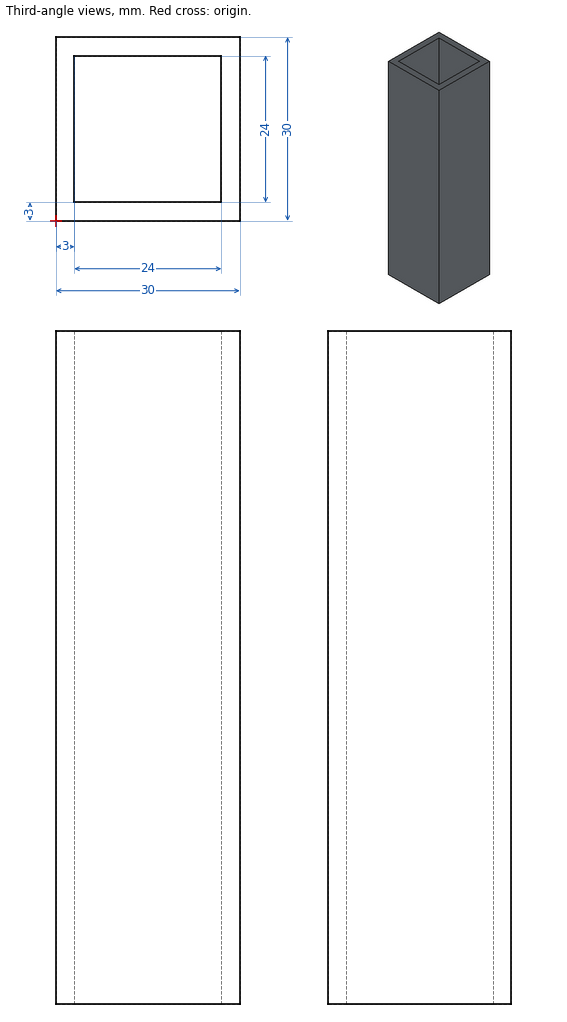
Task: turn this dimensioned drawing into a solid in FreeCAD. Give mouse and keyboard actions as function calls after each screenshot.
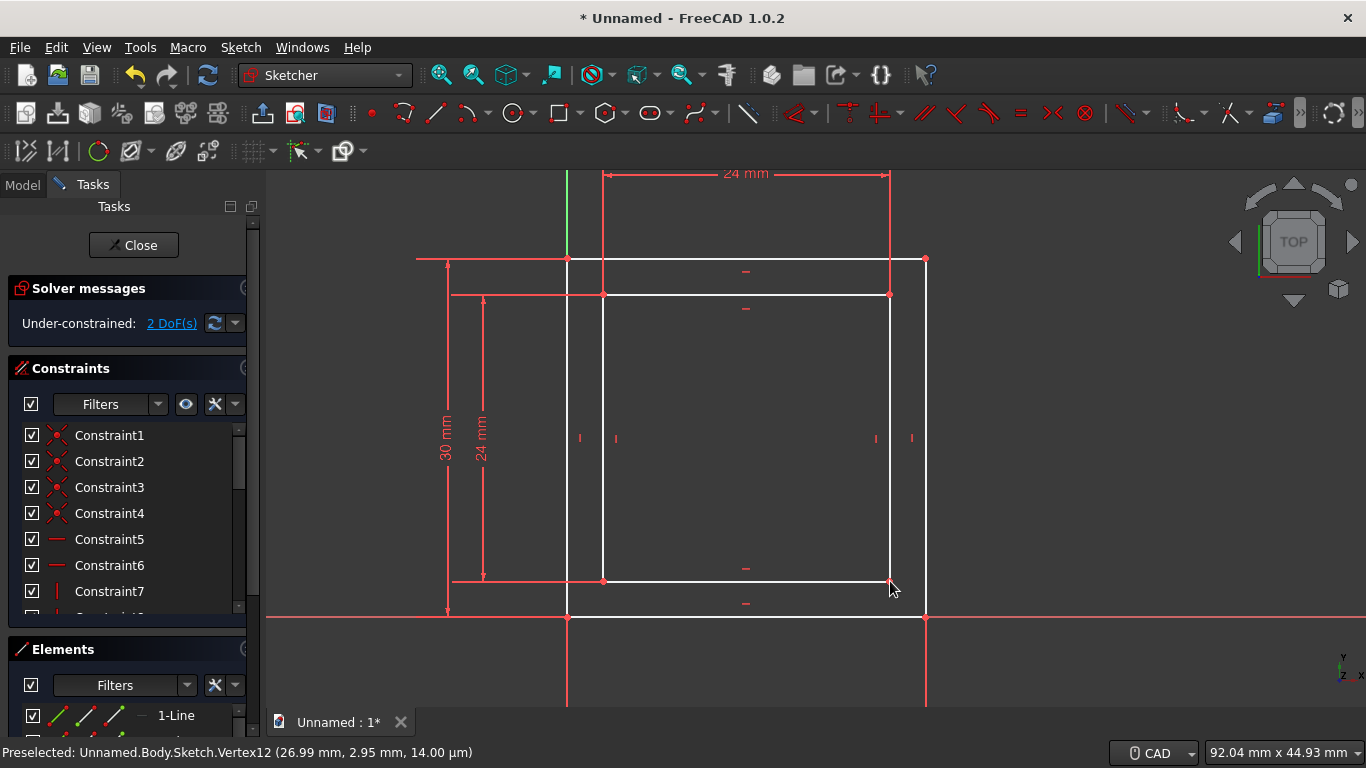
click(794, 114)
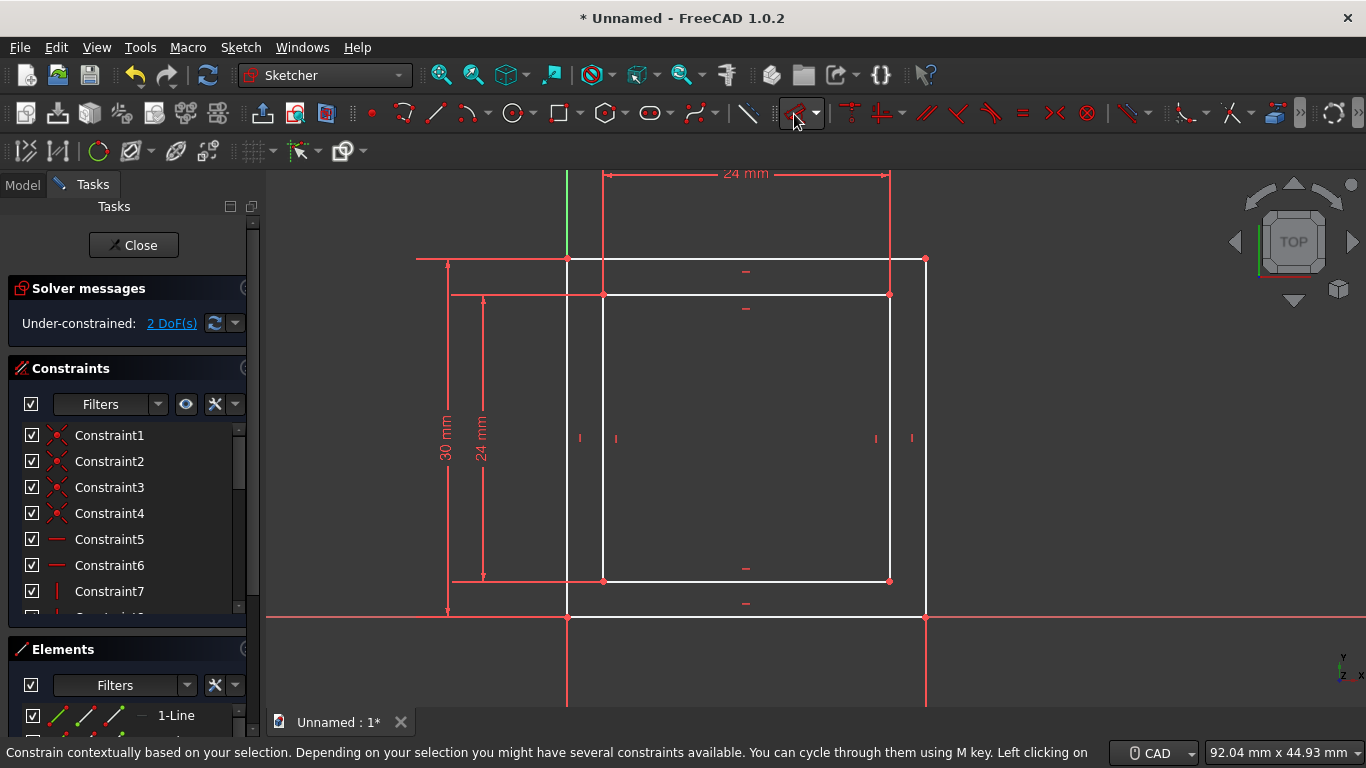
click(603, 295)
click(585, 651)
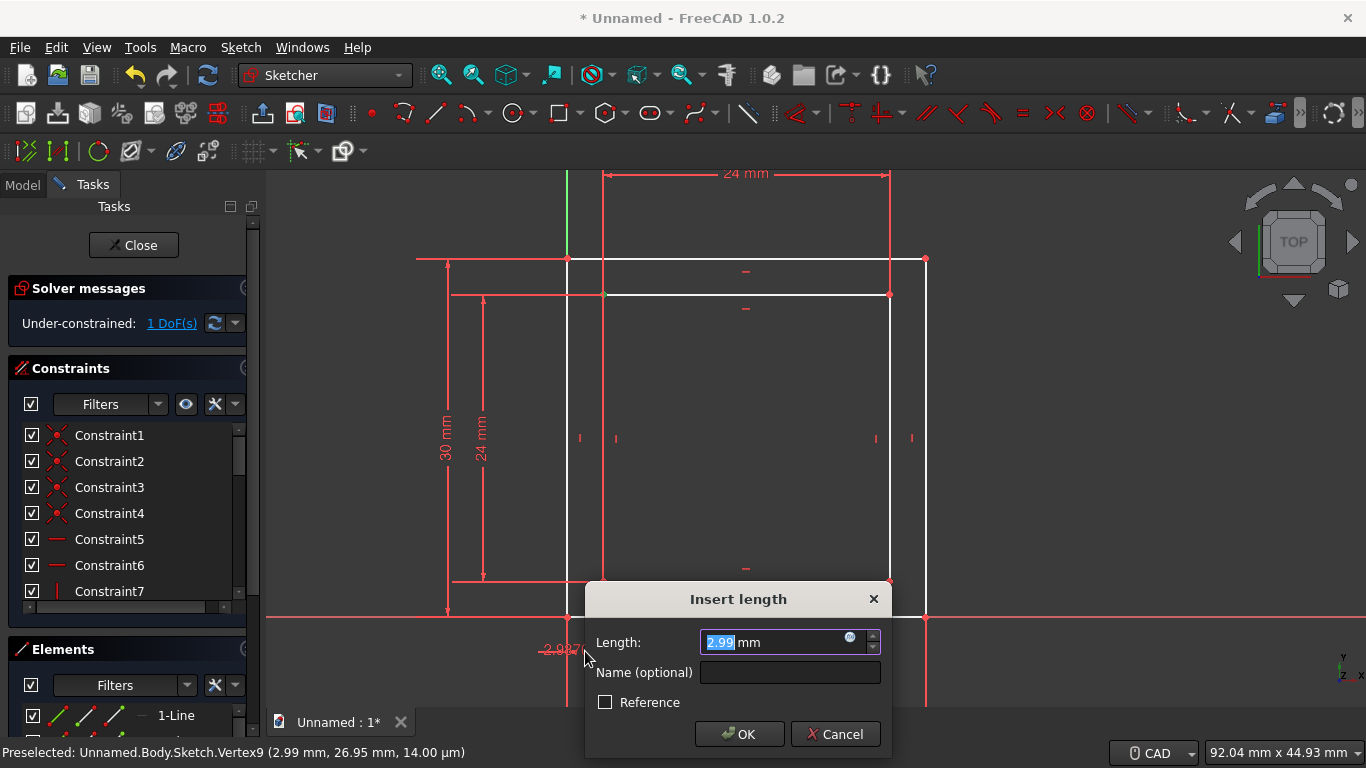
text(3)
key(Return)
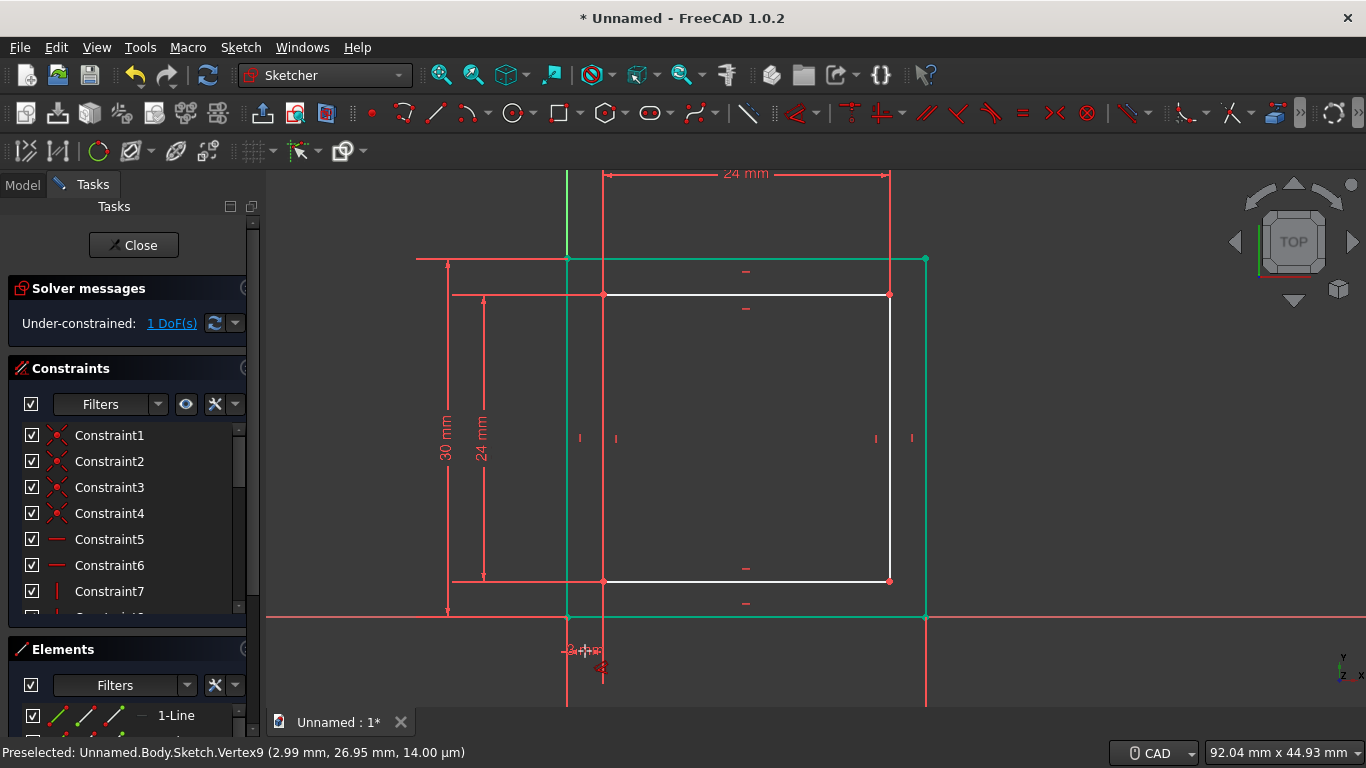
click(603, 582)
click(533, 599)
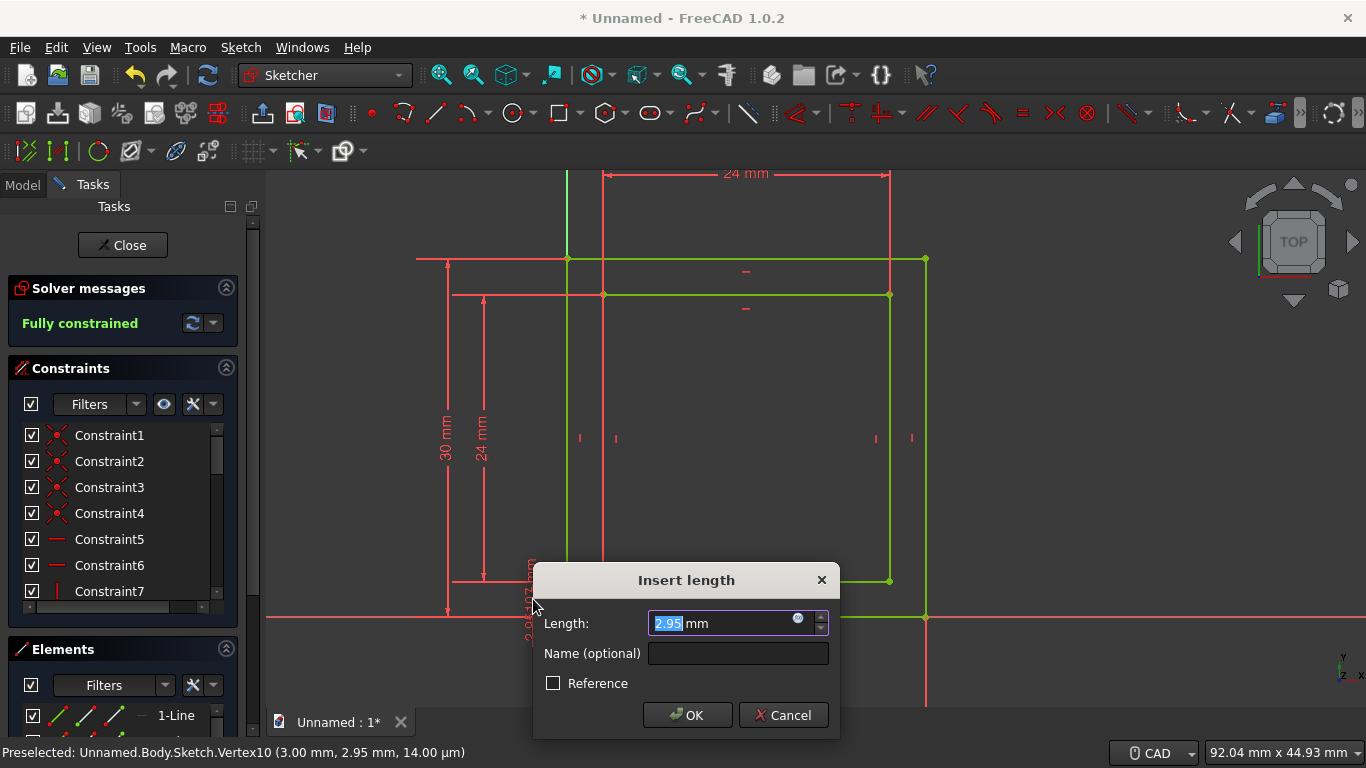
text(3)
key(Return)
key(Escape)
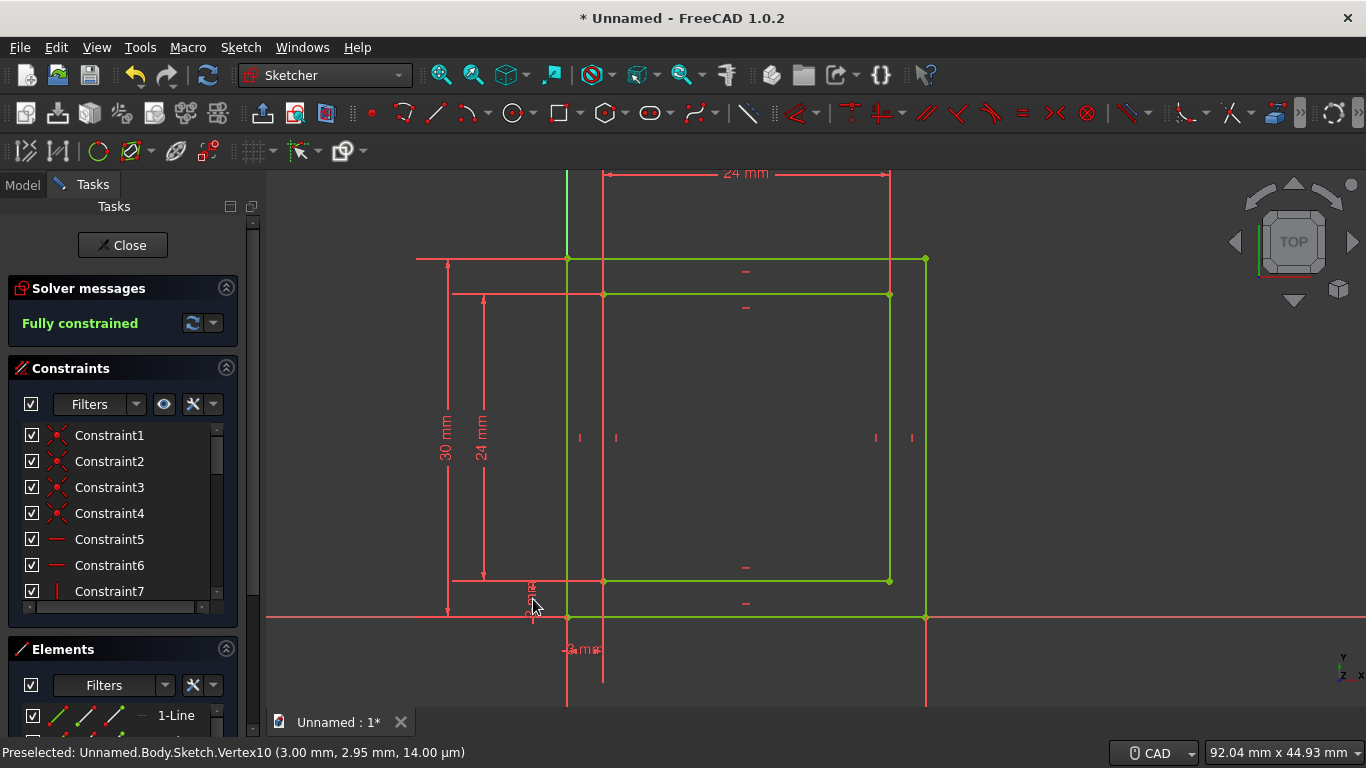
click(123, 245)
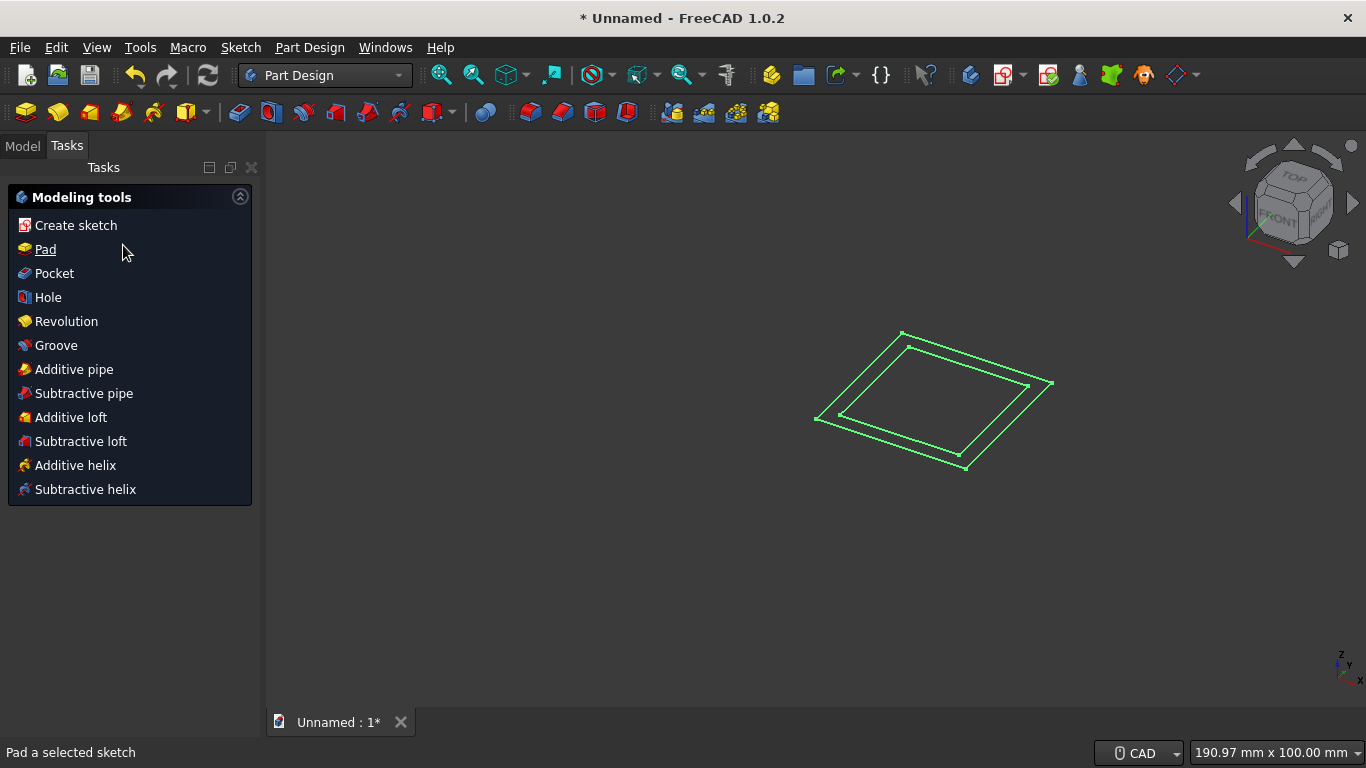
click(26, 112)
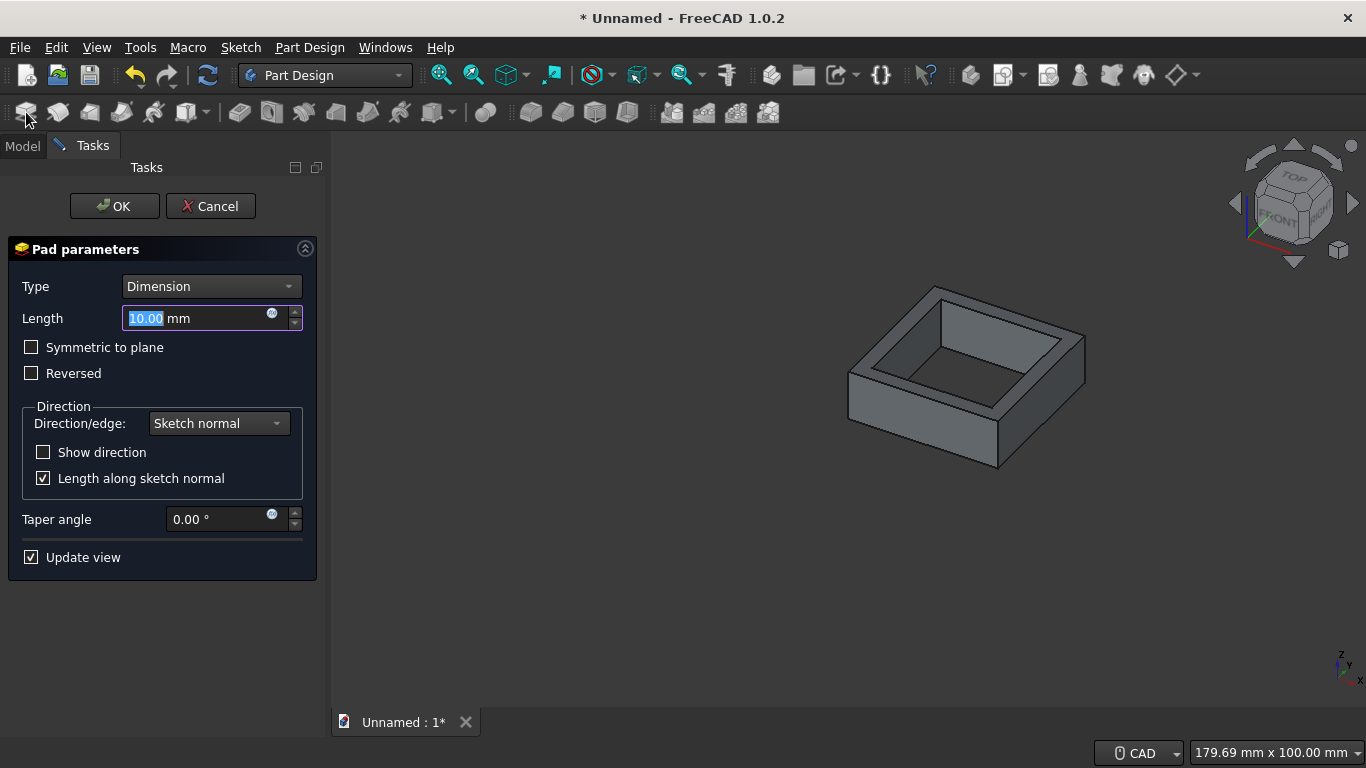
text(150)
key(Tab)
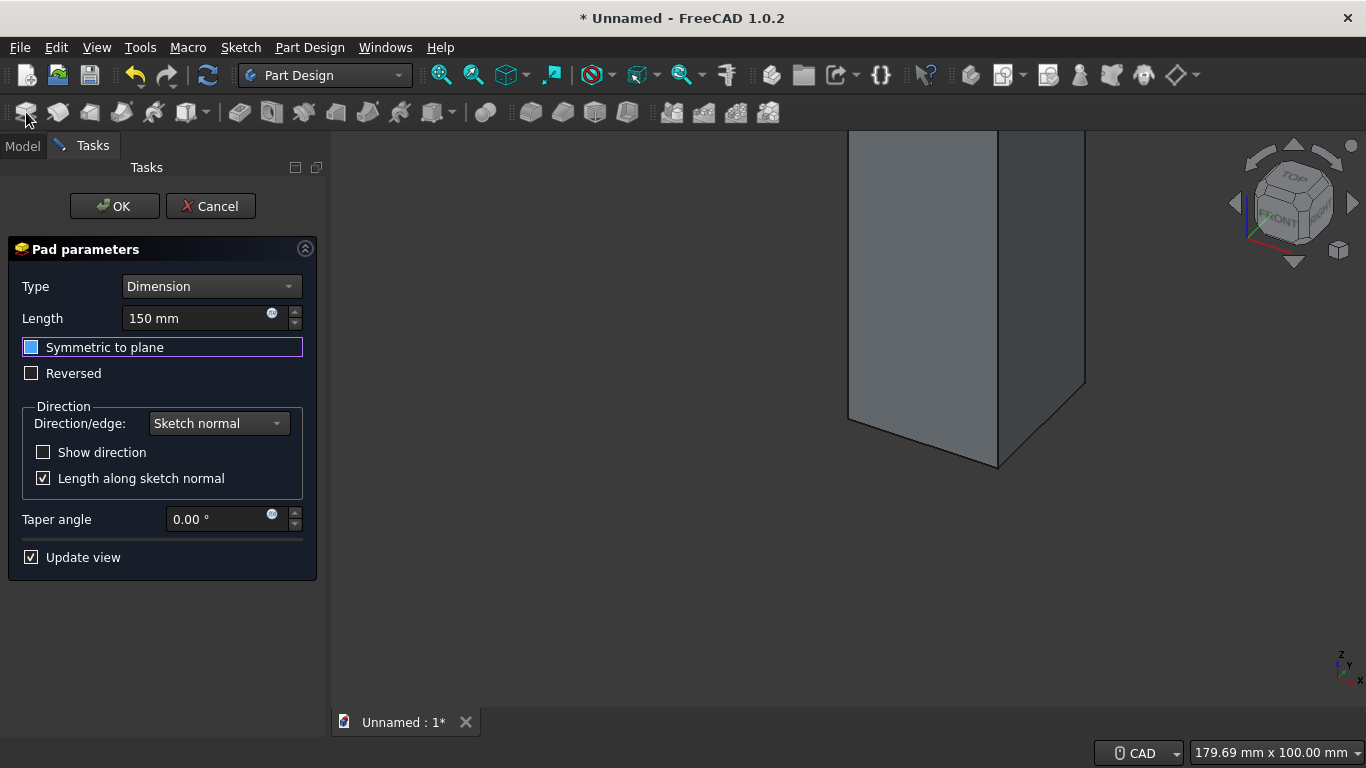
click(115, 206)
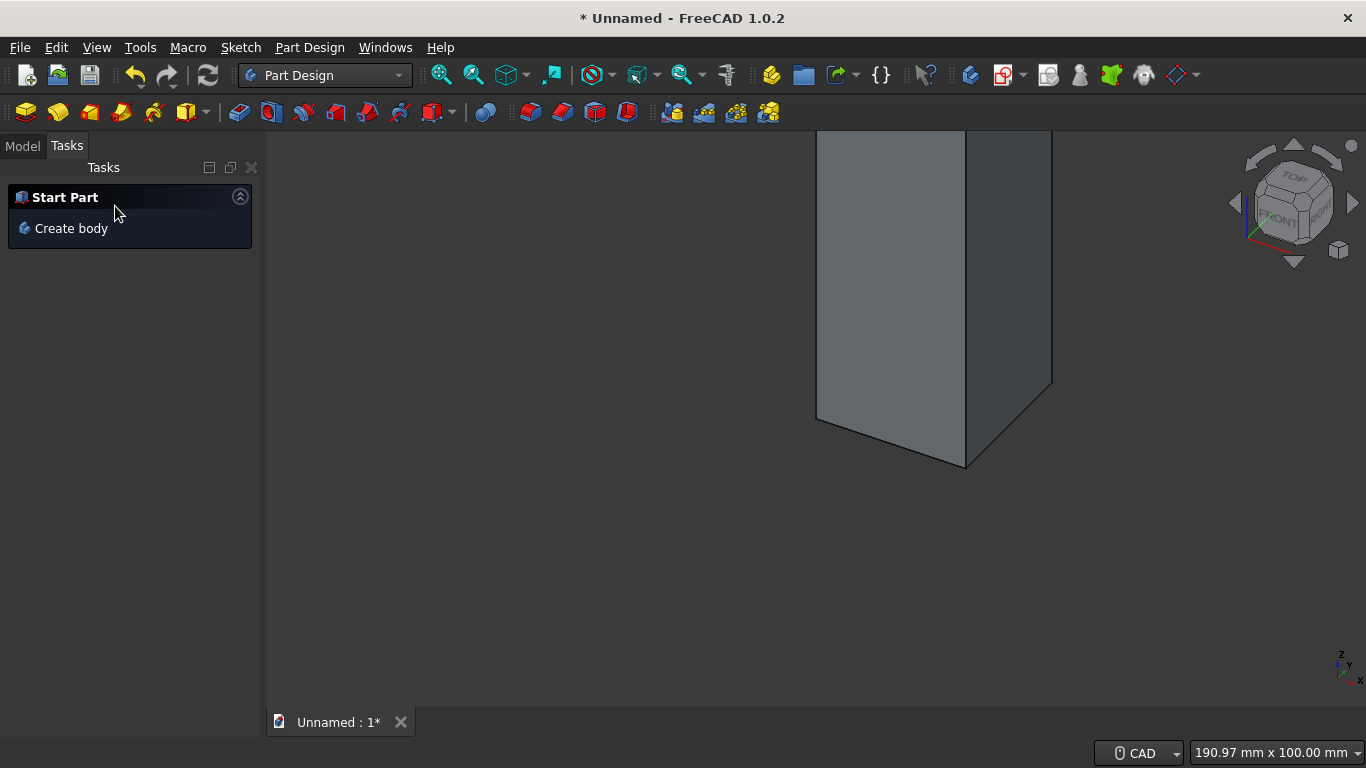
click(442, 76)